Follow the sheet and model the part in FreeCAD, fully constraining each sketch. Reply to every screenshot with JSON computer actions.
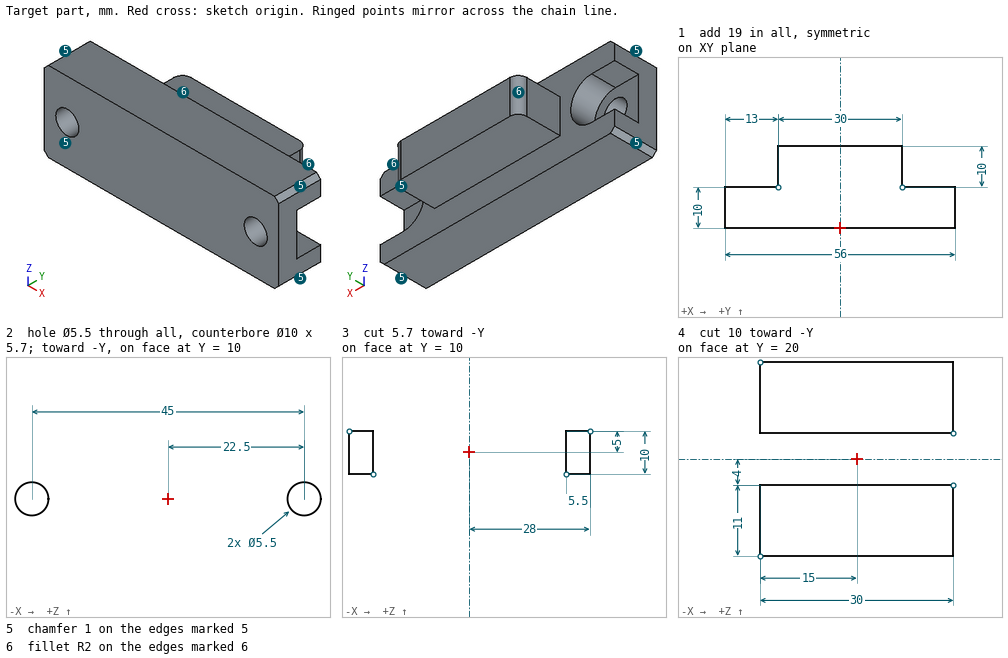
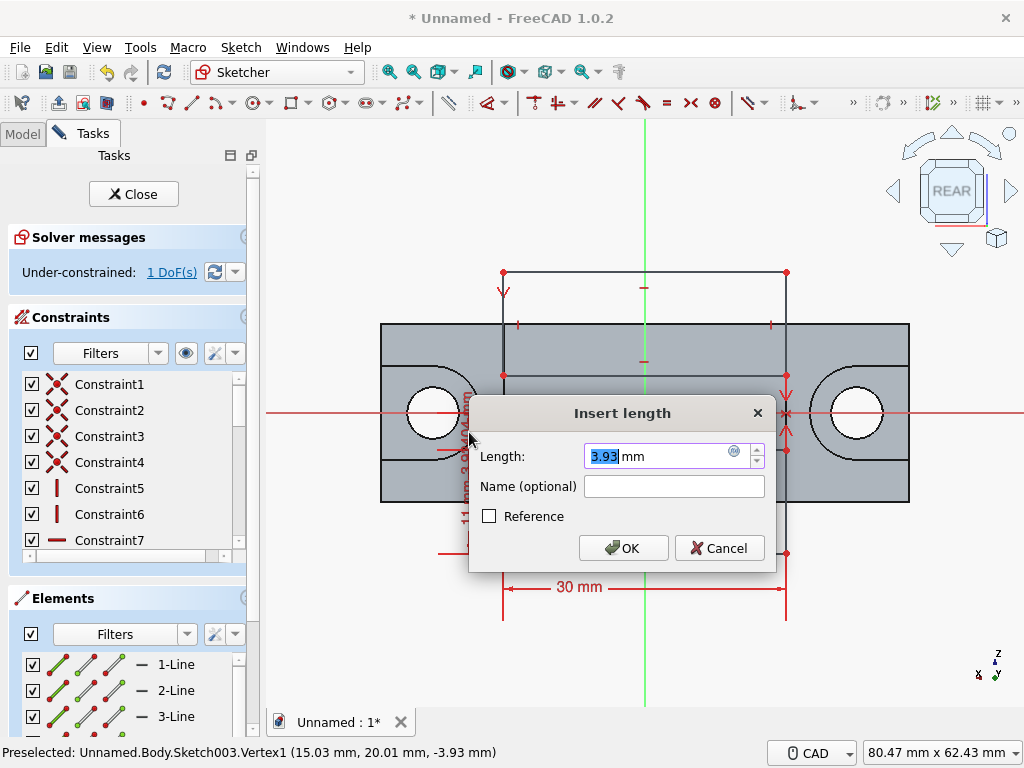
{"action": "type", "text": "4"}
{"action": "key", "text": "Return"}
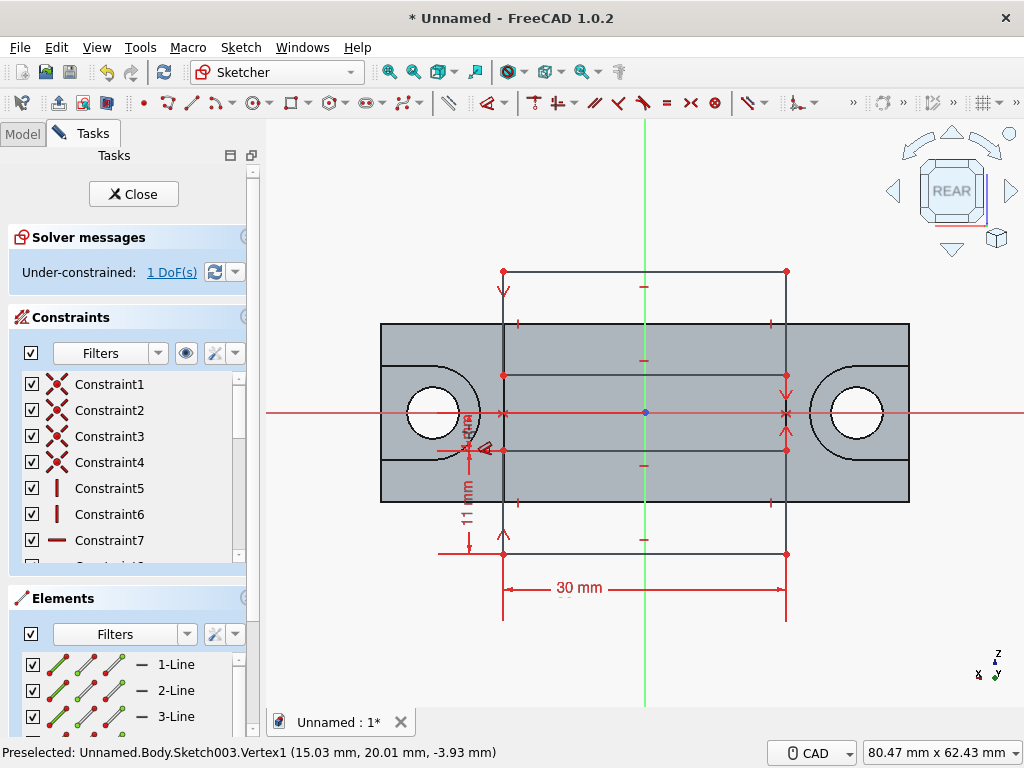
{"action": "left_click", "coordinate": [503, 451]}
{"action": "left_click", "coordinate": [574, 485]}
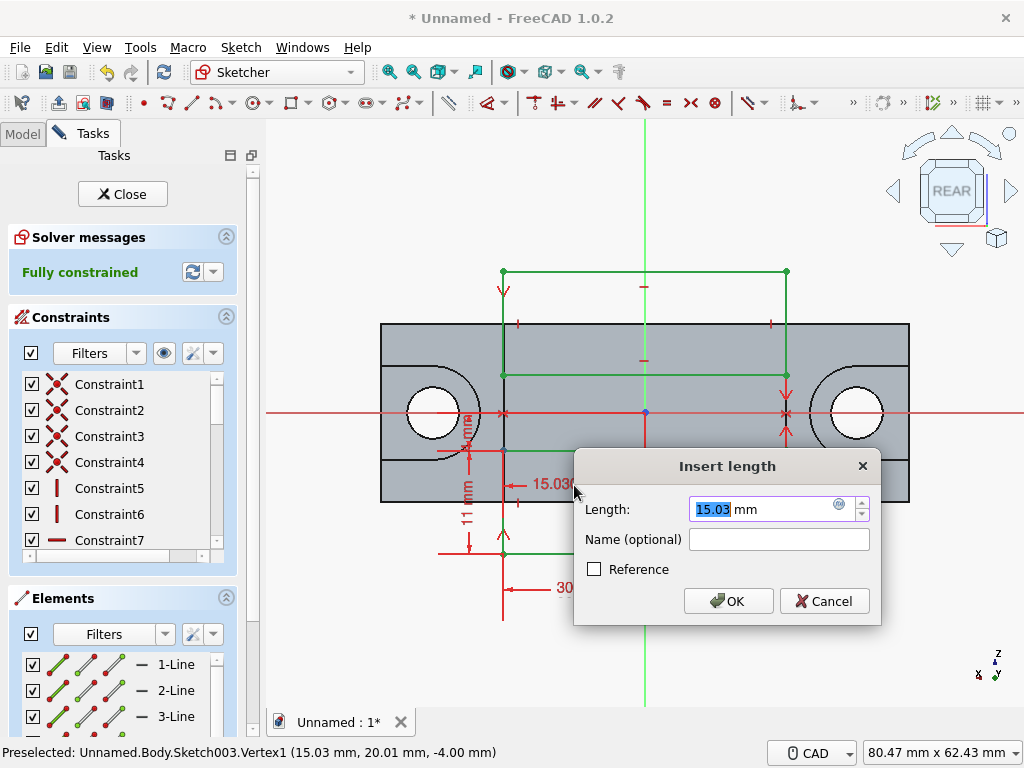
{"action": "type", "text": "15"}
{"action": "key", "text": "Return"}
{"action": "key", "text": "Escape"}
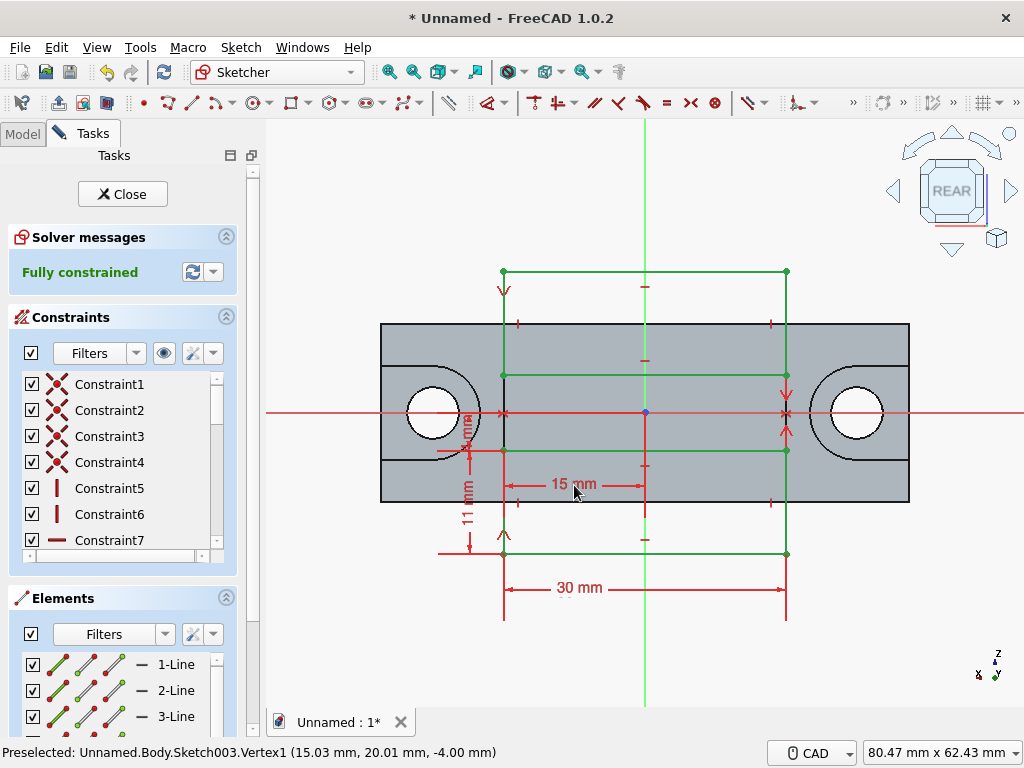
{"action": "left_click", "coordinate": [123, 194]}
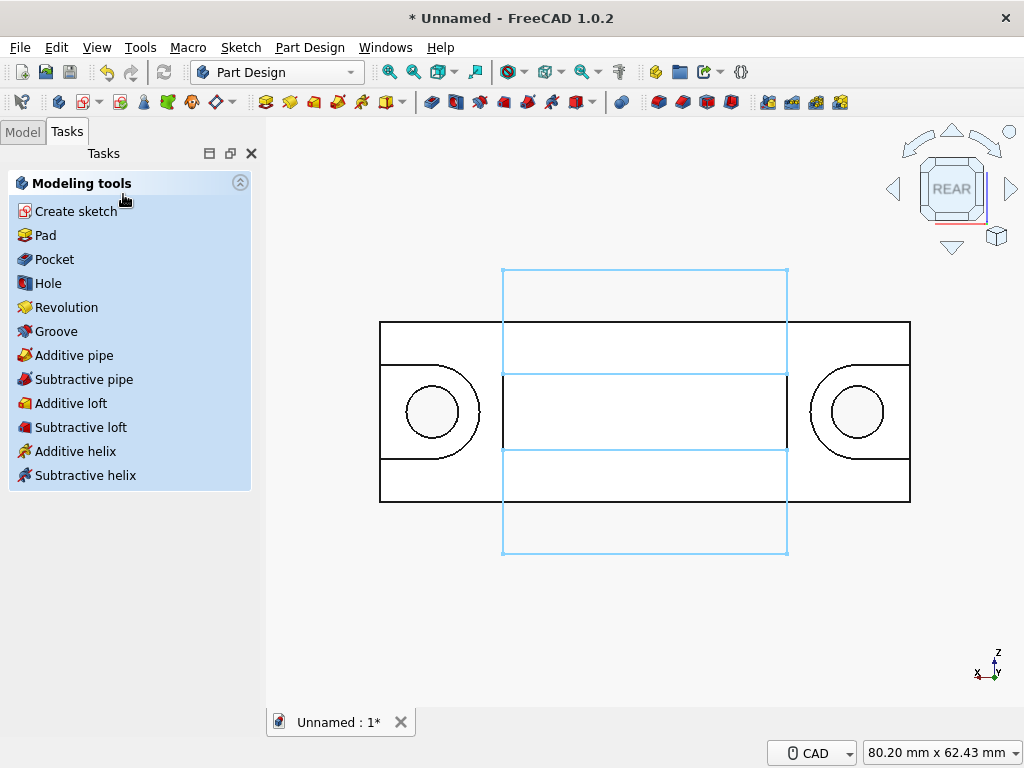
{"action": "left_click", "coordinate": [432, 102]}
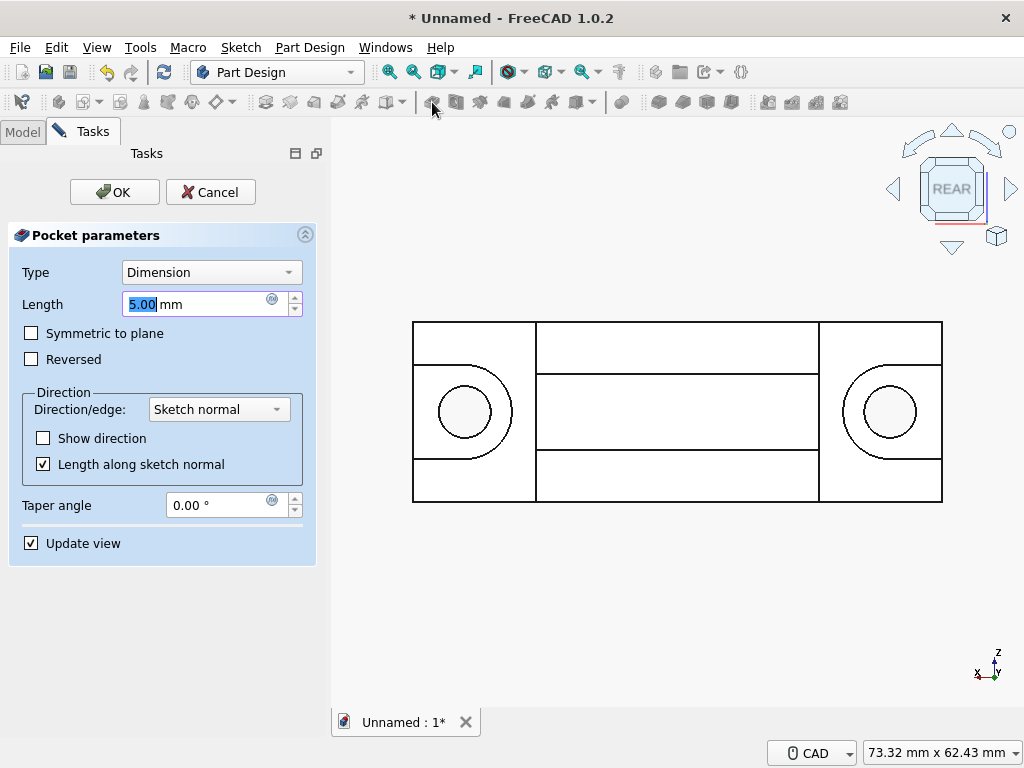
{"action": "type", "text": "10"}
{"action": "key", "text": "Tab"}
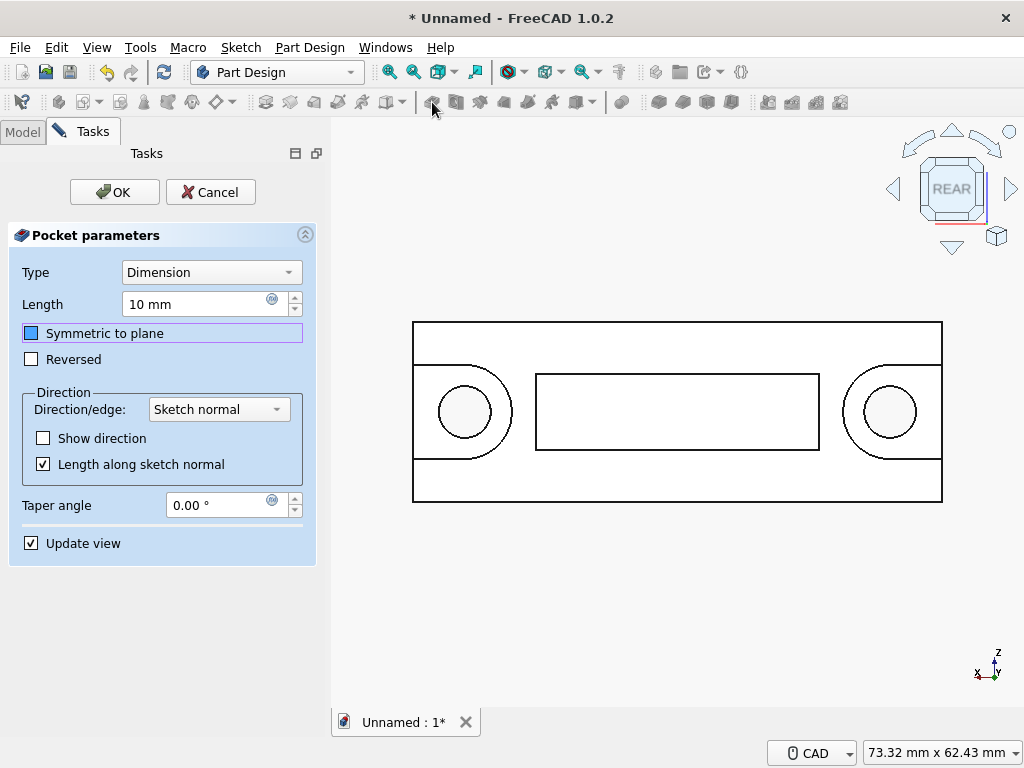
{"action": "left_click", "coordinate": [115, 192]}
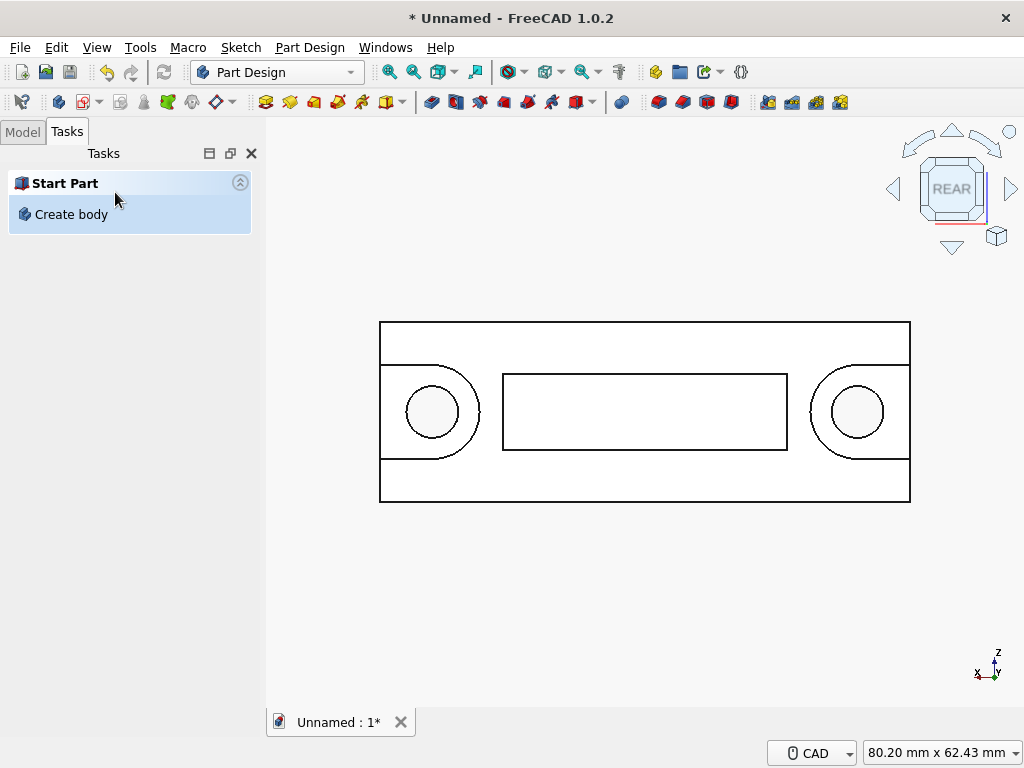
{"action": "key", "text": "0"}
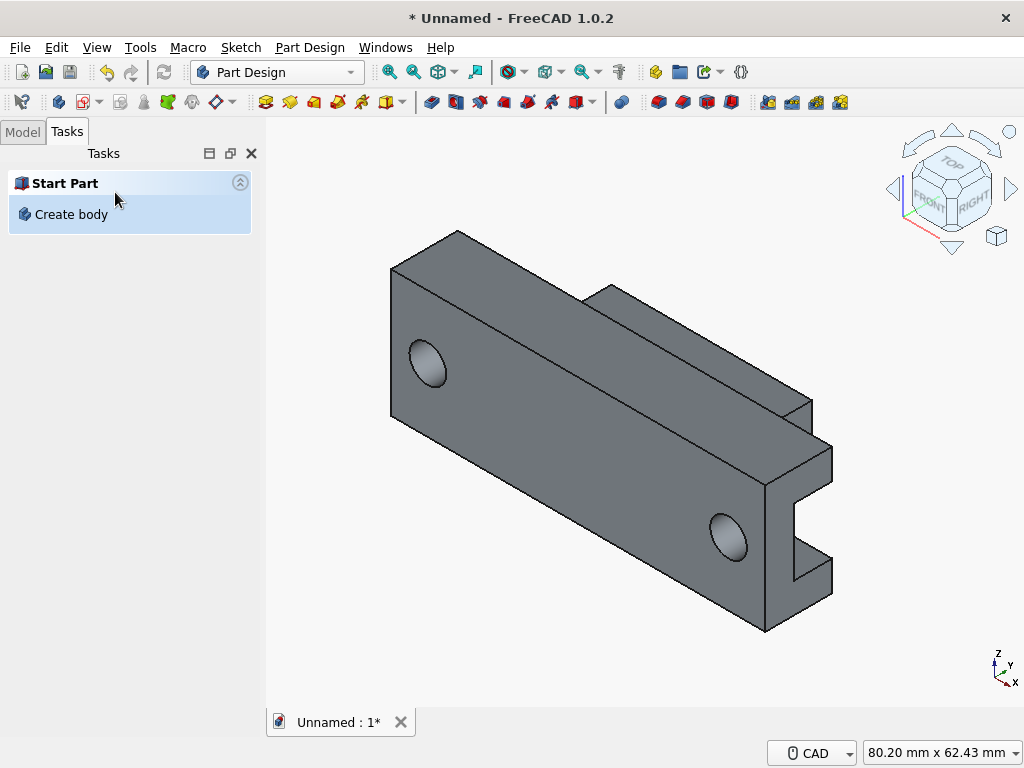
{"action": "left_click", "coordinate": [799, 465]}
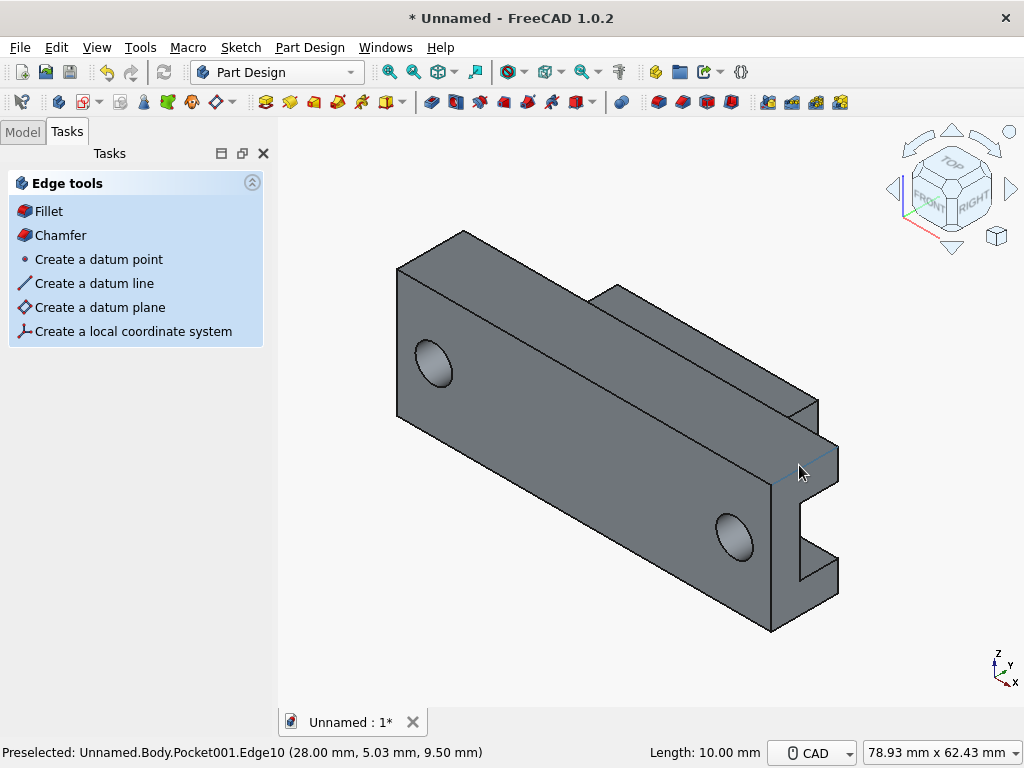
{"action": "key", "text": "2"}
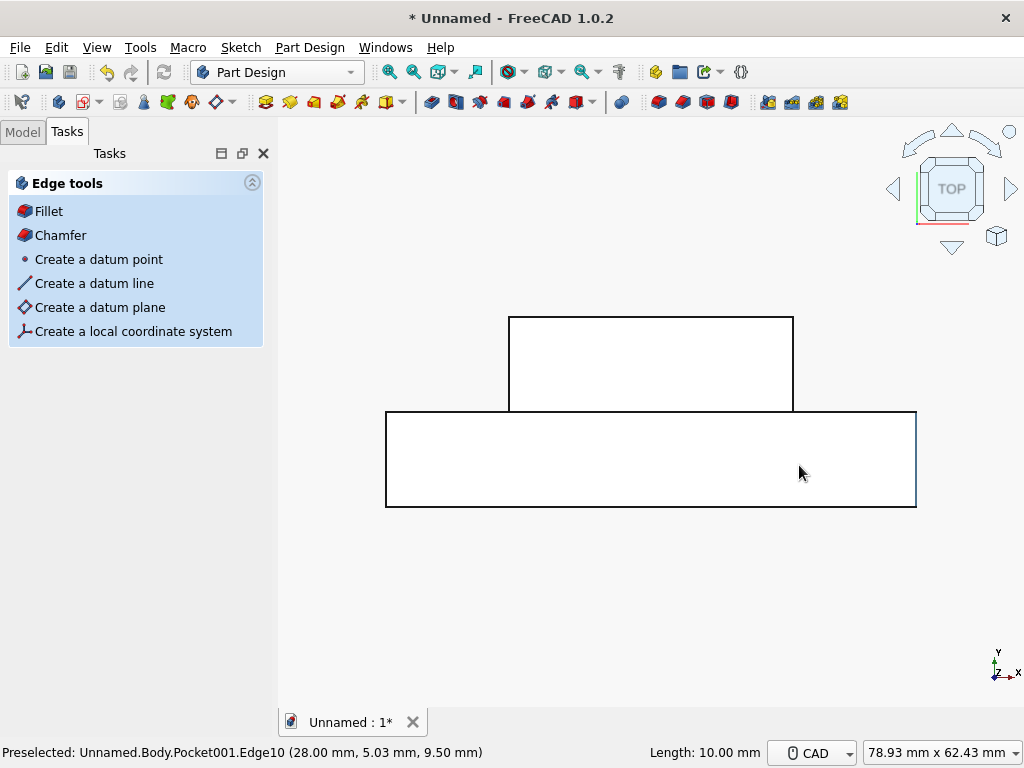
{"action": "left_click", "coordinate": [386, 458], "text": "ctrl"}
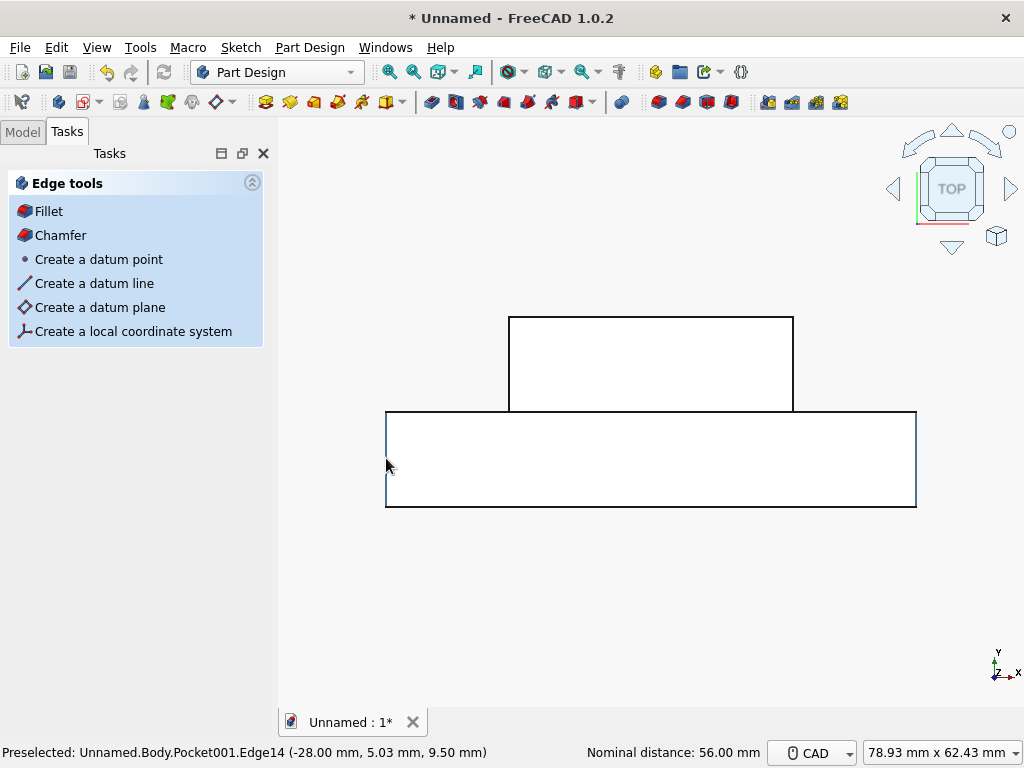
{"action": "key", "text": "1"}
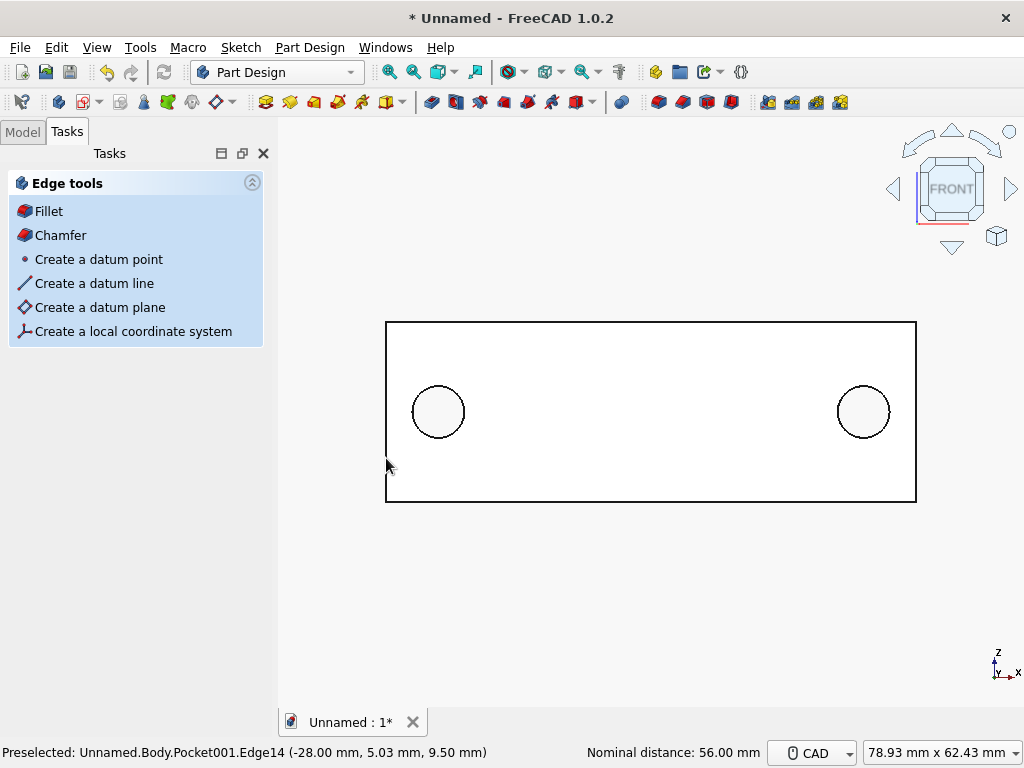
{"action": "key", "text": "3"}